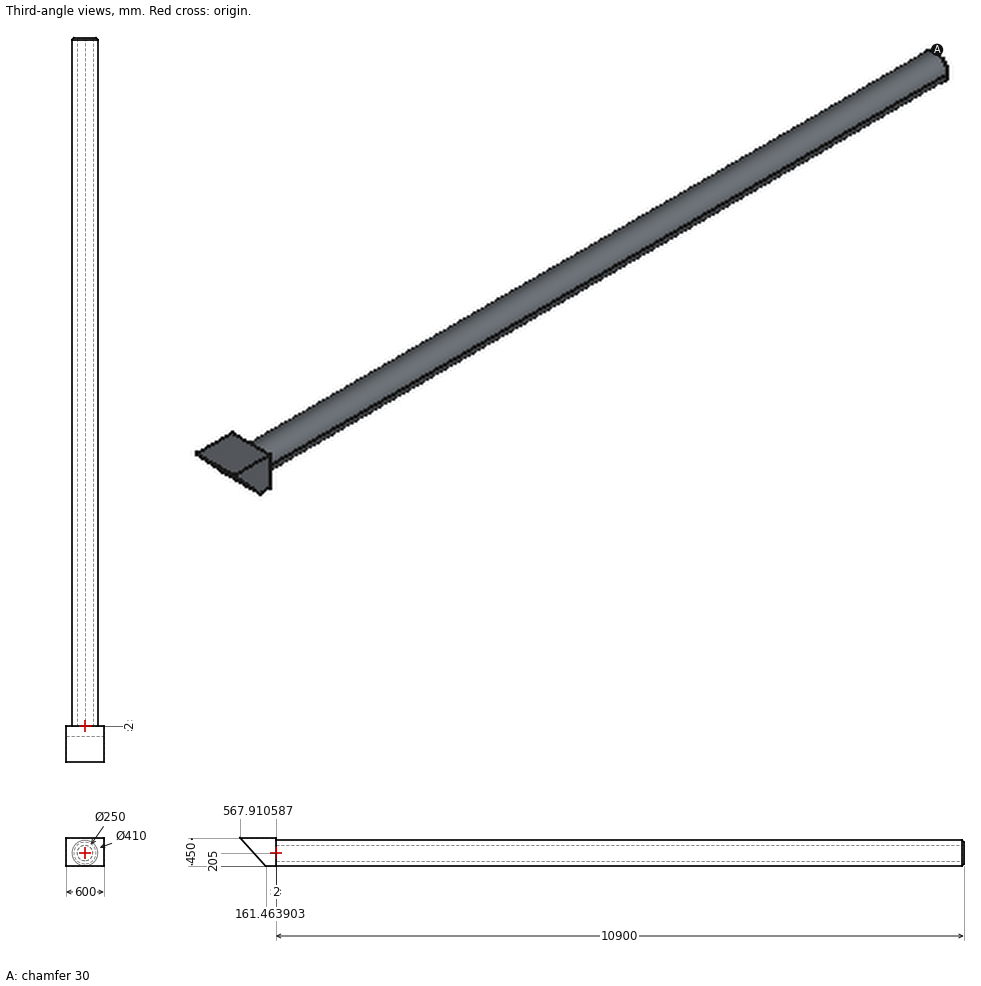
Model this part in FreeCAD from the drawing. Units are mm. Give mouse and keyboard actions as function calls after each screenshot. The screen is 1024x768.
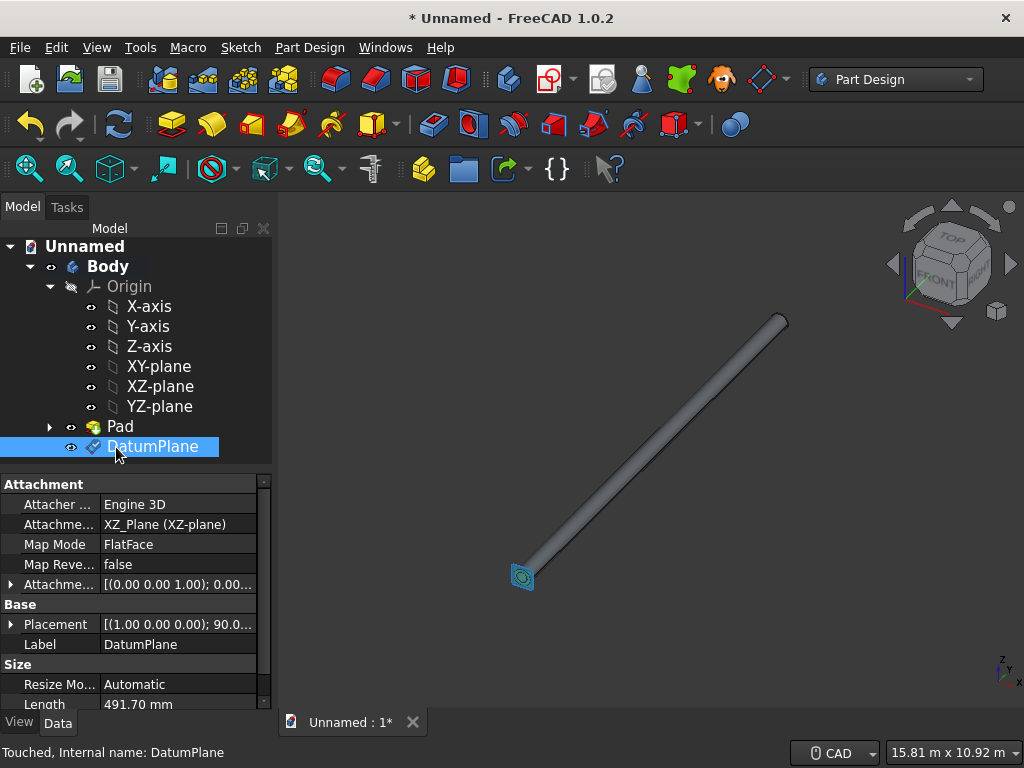
click(550, 80)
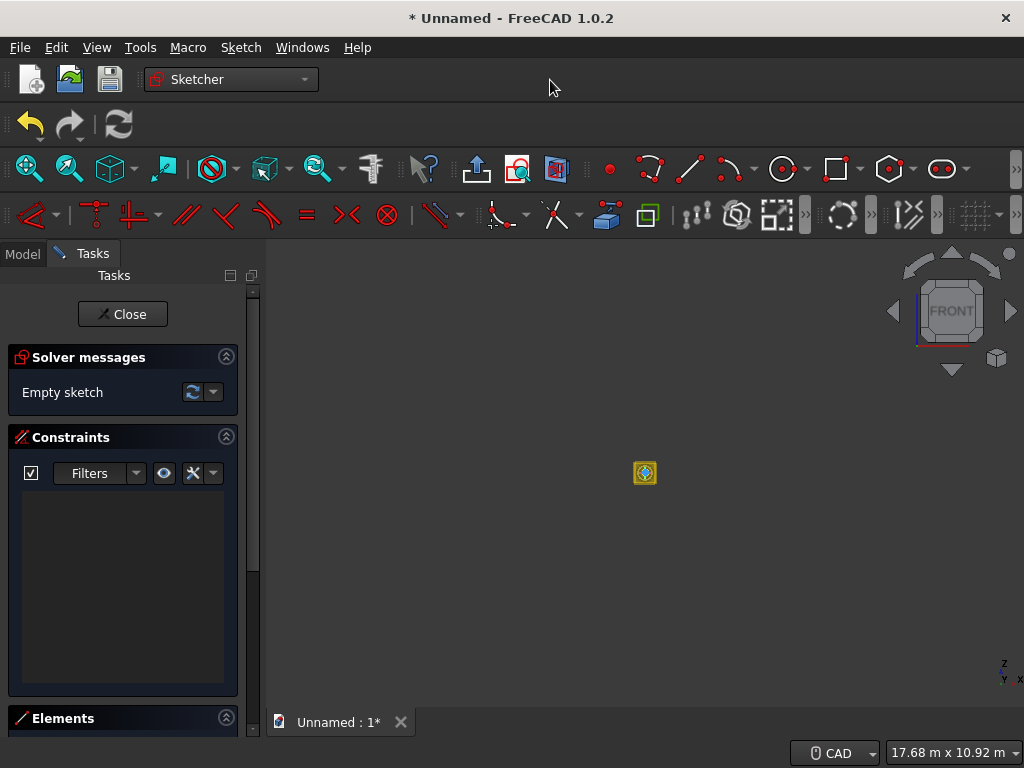
scroll(649, 473, up, 14)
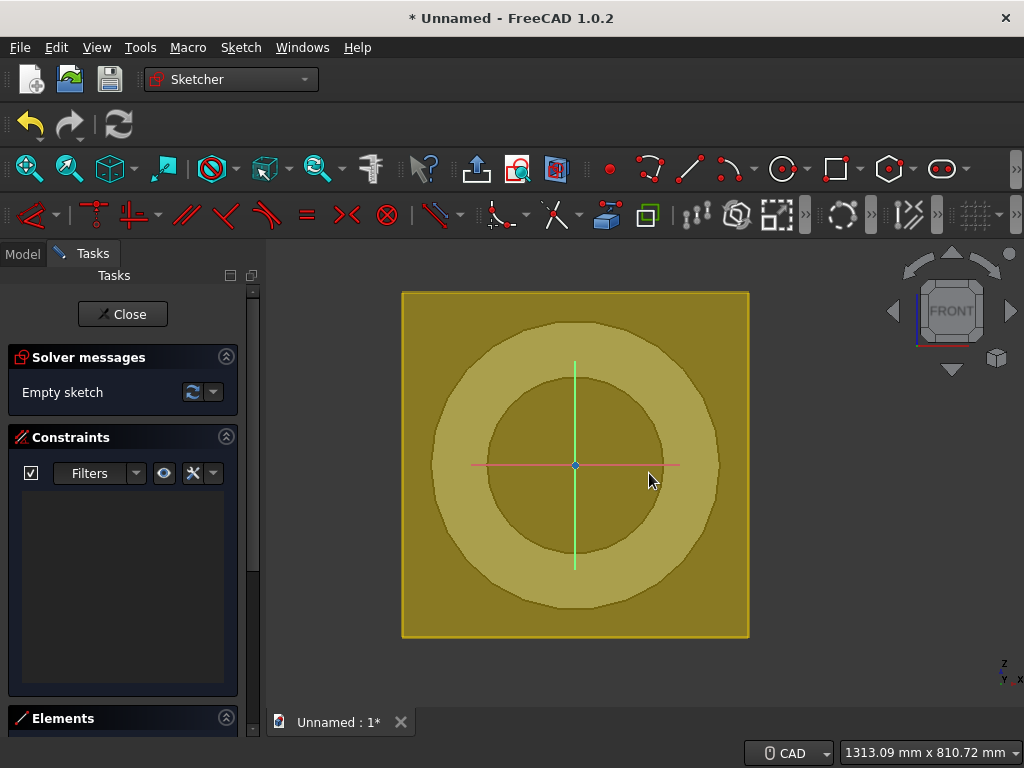
click(784, 170)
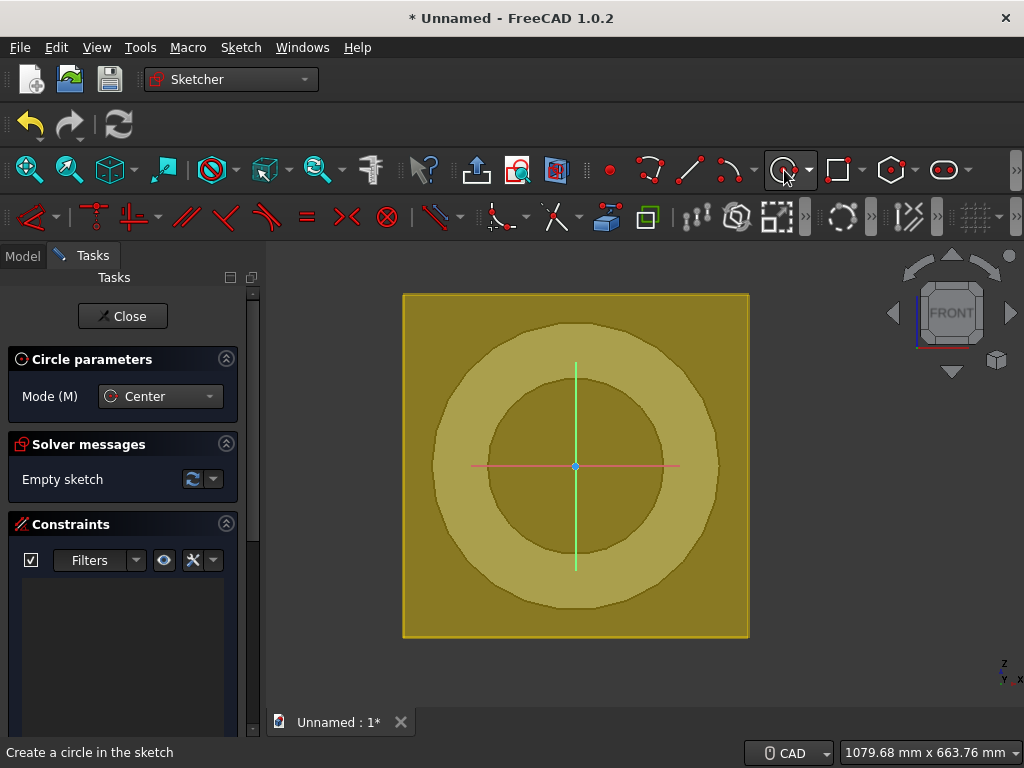
click(576, 466)
move(677, 365)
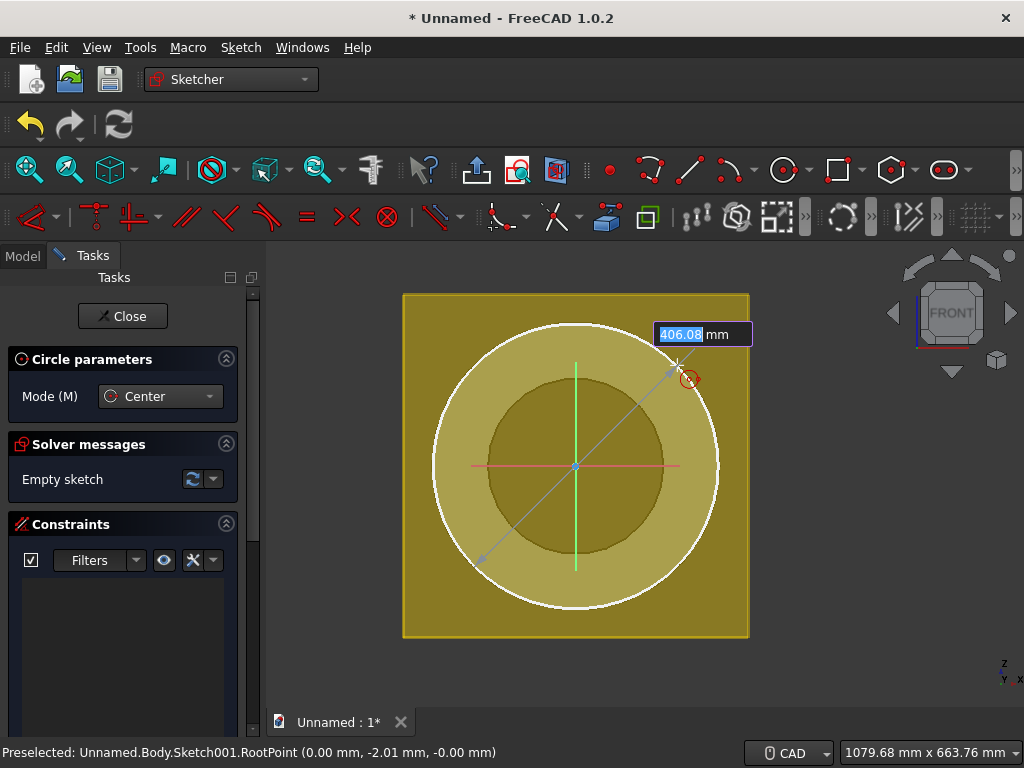
text(410)
key(Return)
key(Escape)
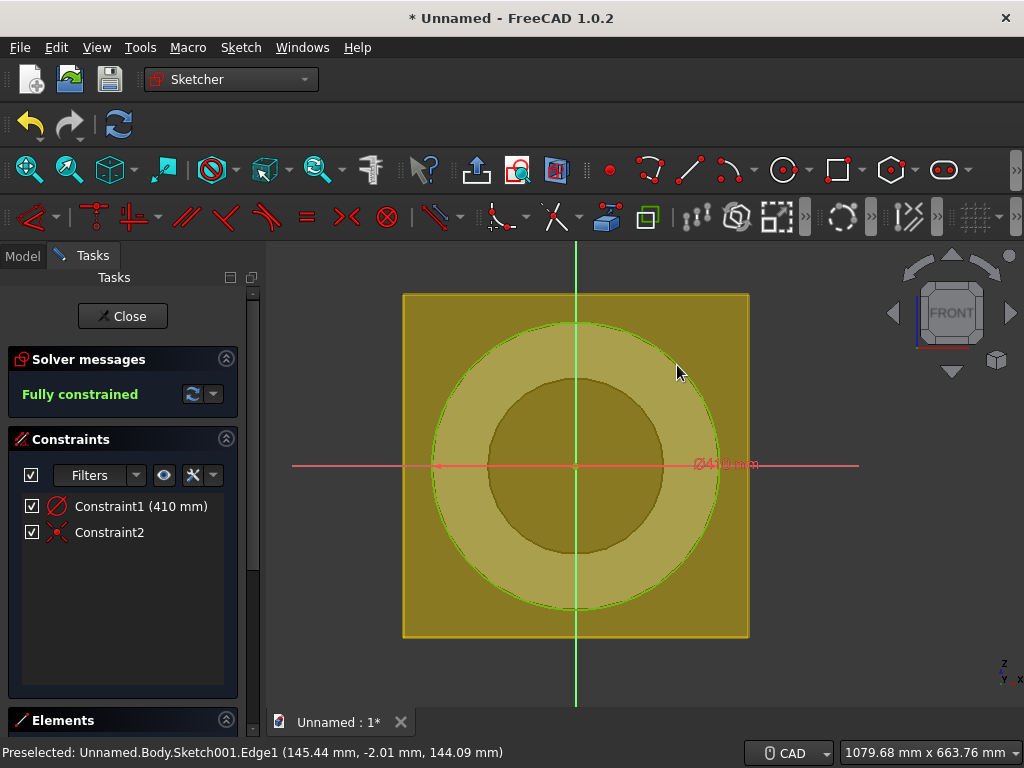
click(123, 316)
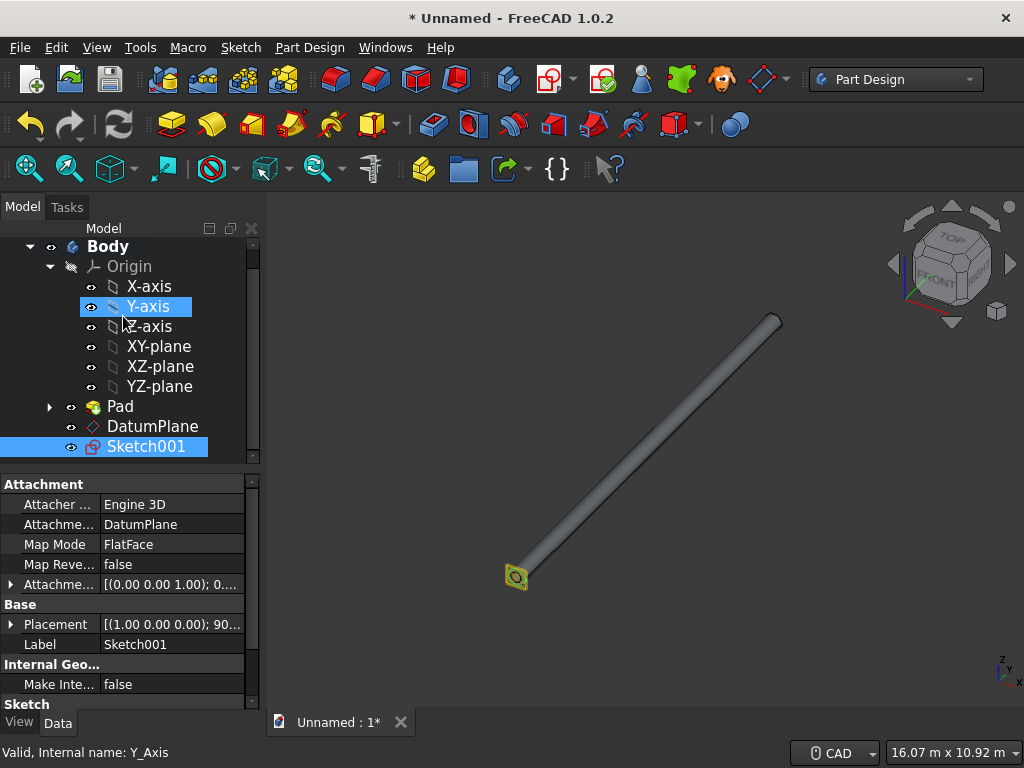
click(172, 124)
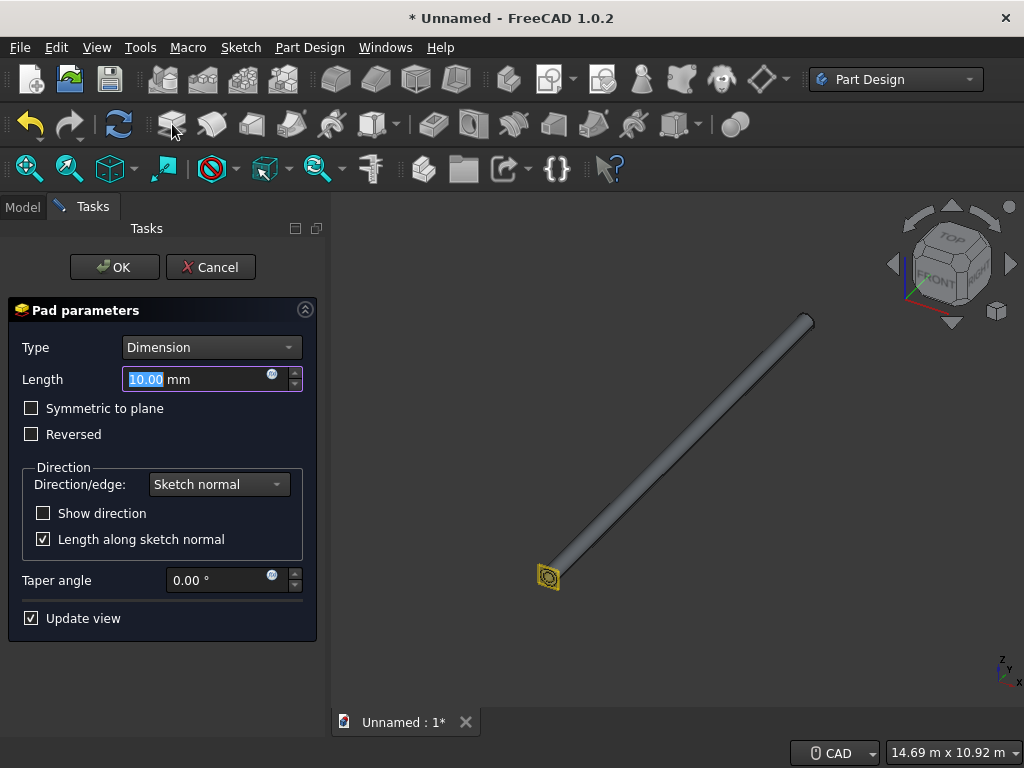
text(2)
key(Tab)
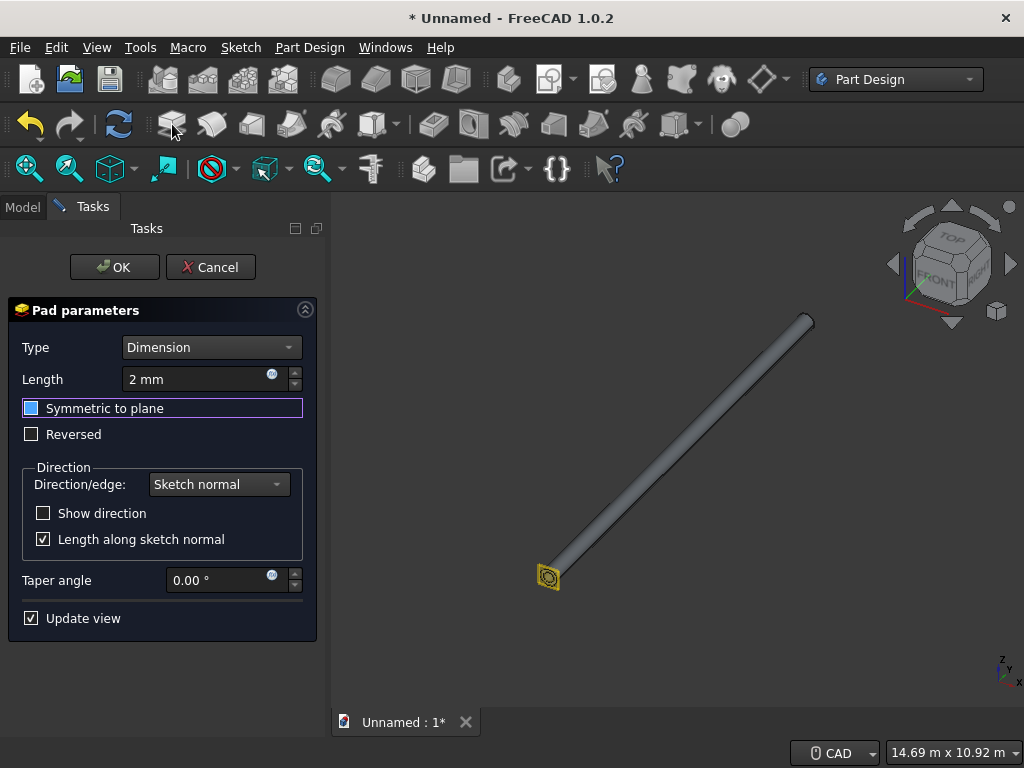
click(30, 434)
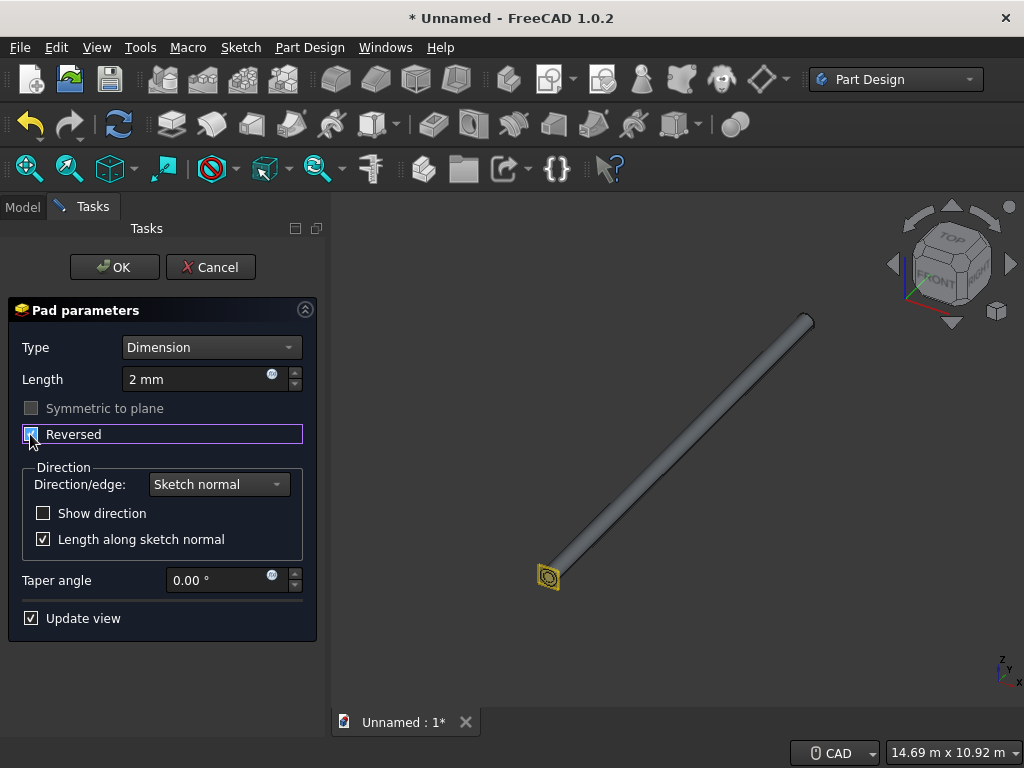
click(115, 267)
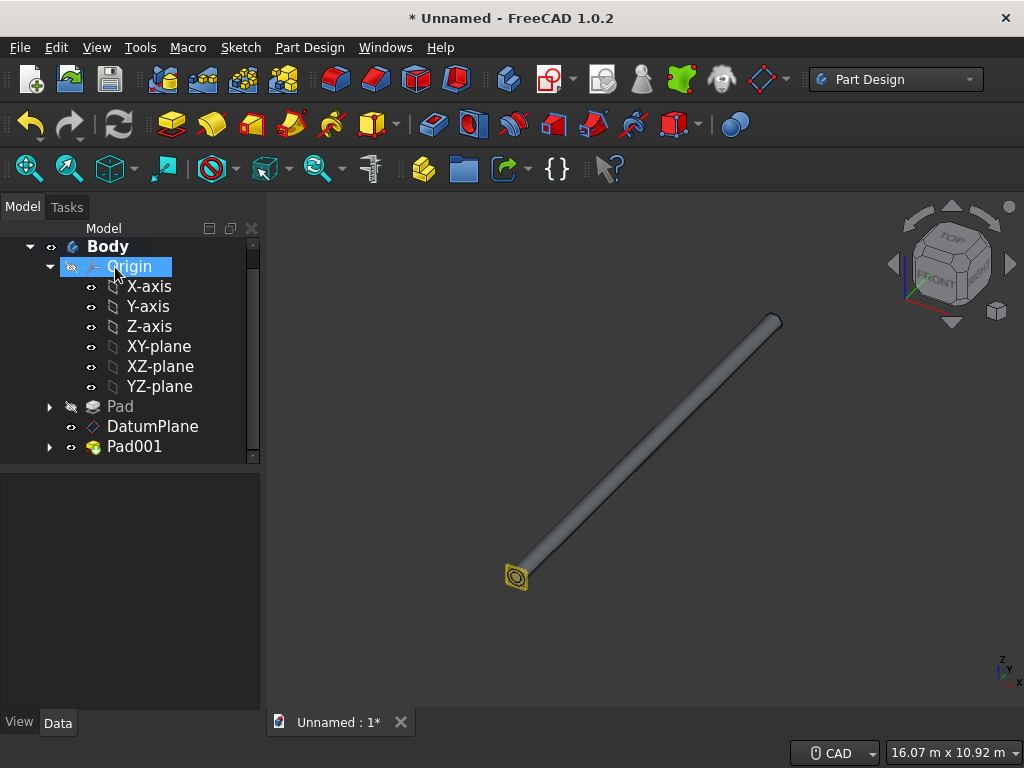
click(116, 427)
key(space)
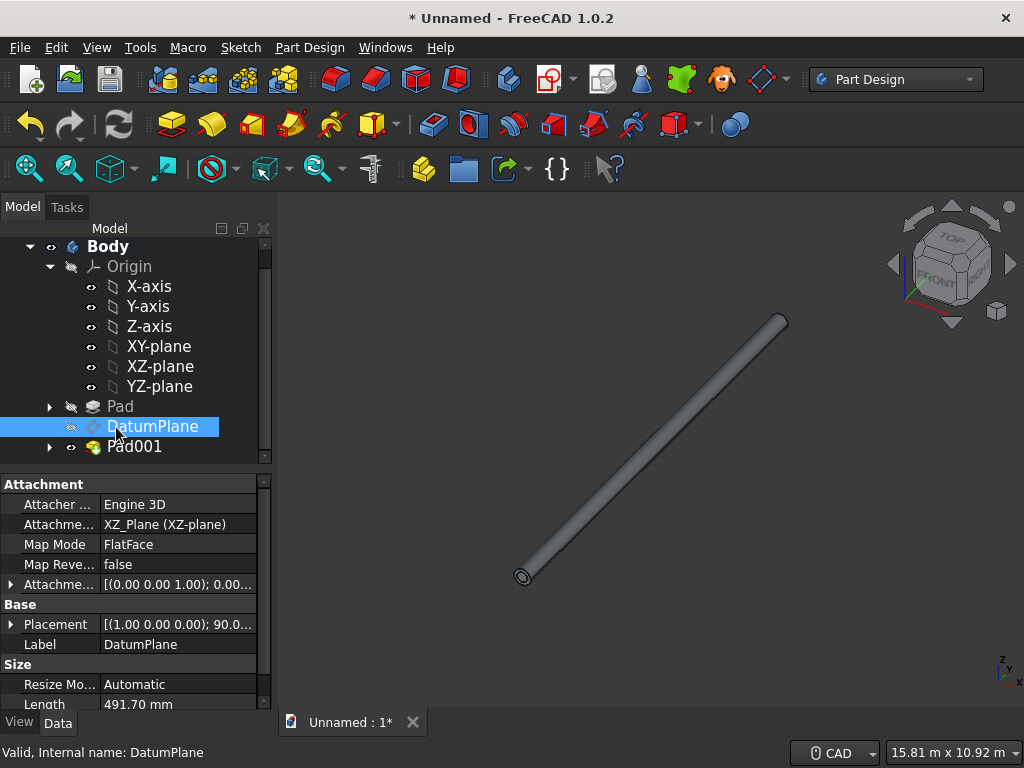
click(777, 312)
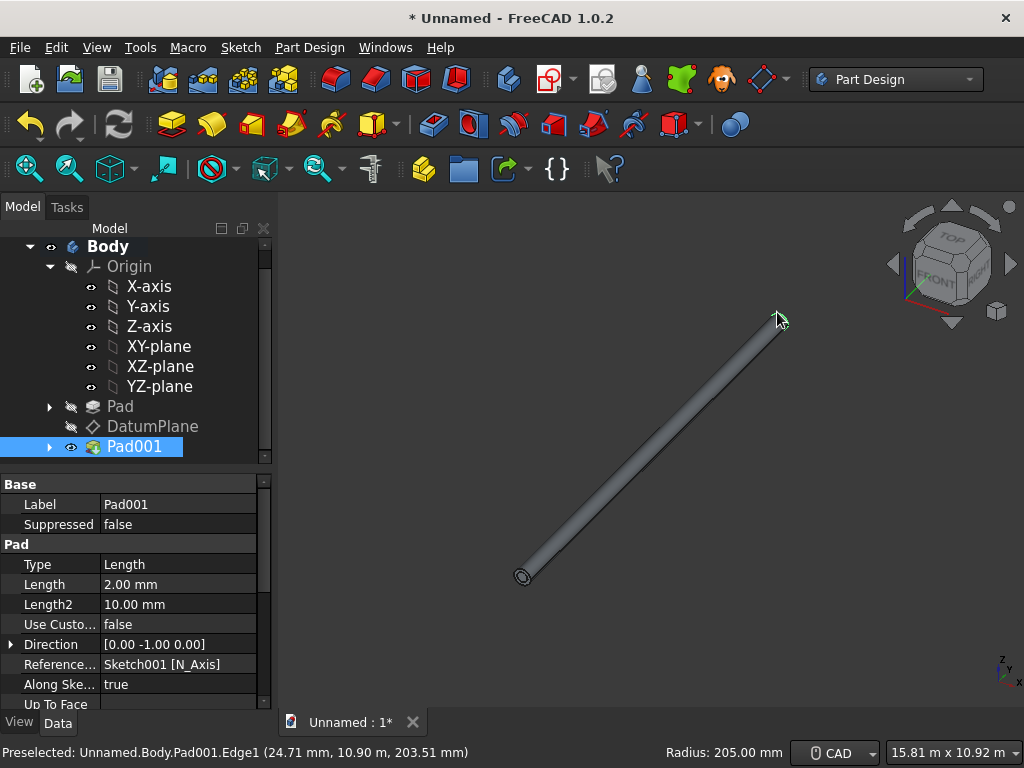
click(376, 80)